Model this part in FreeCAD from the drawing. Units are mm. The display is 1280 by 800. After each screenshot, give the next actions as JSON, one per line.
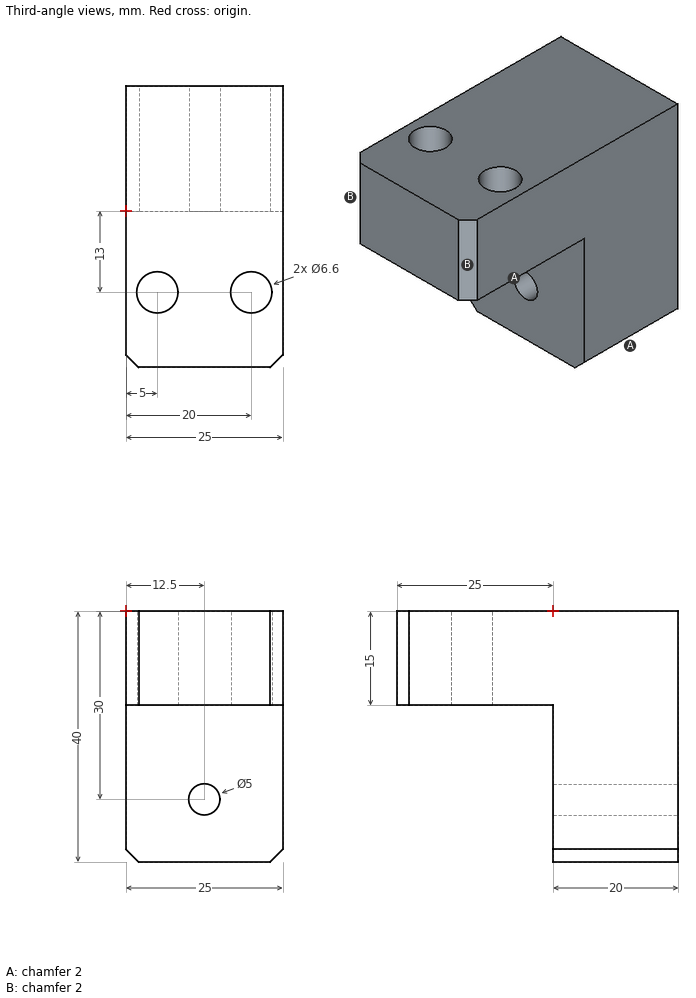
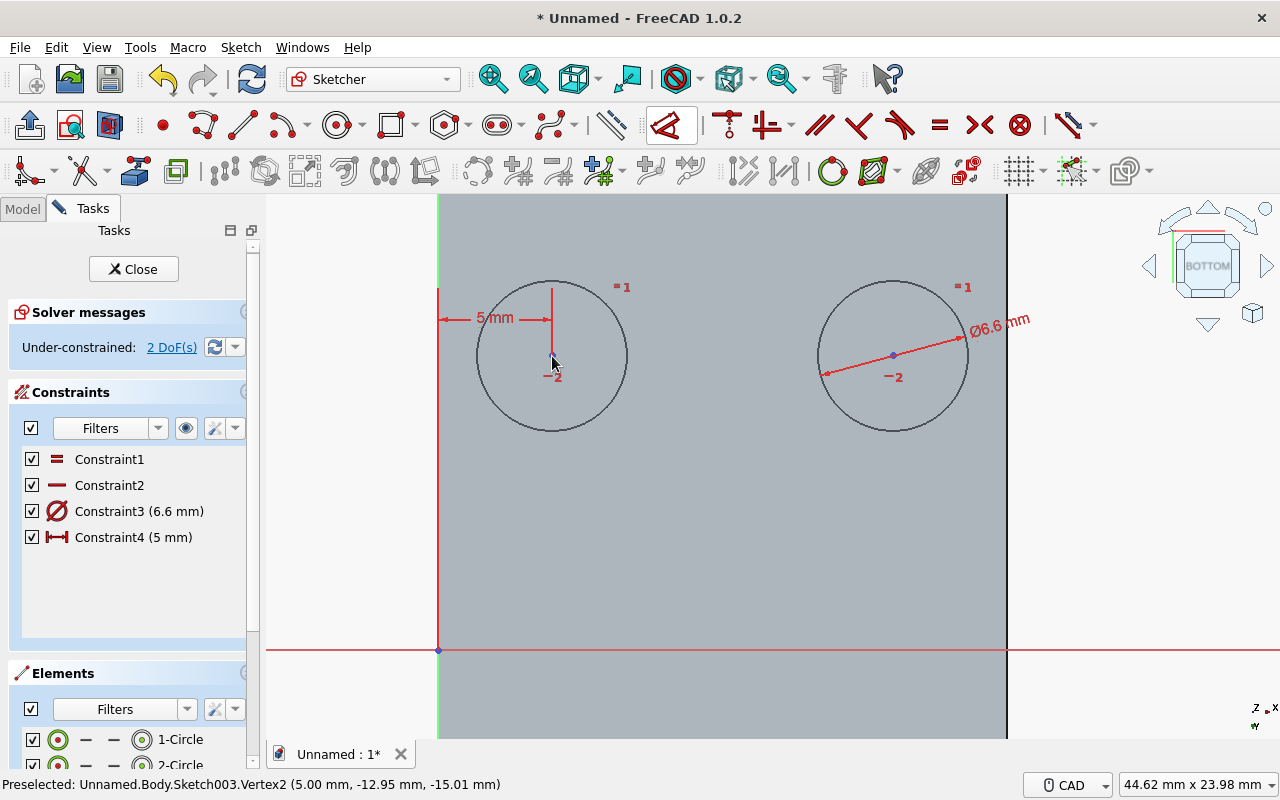
{"action": "left_click", "coordinate": [893, 356]}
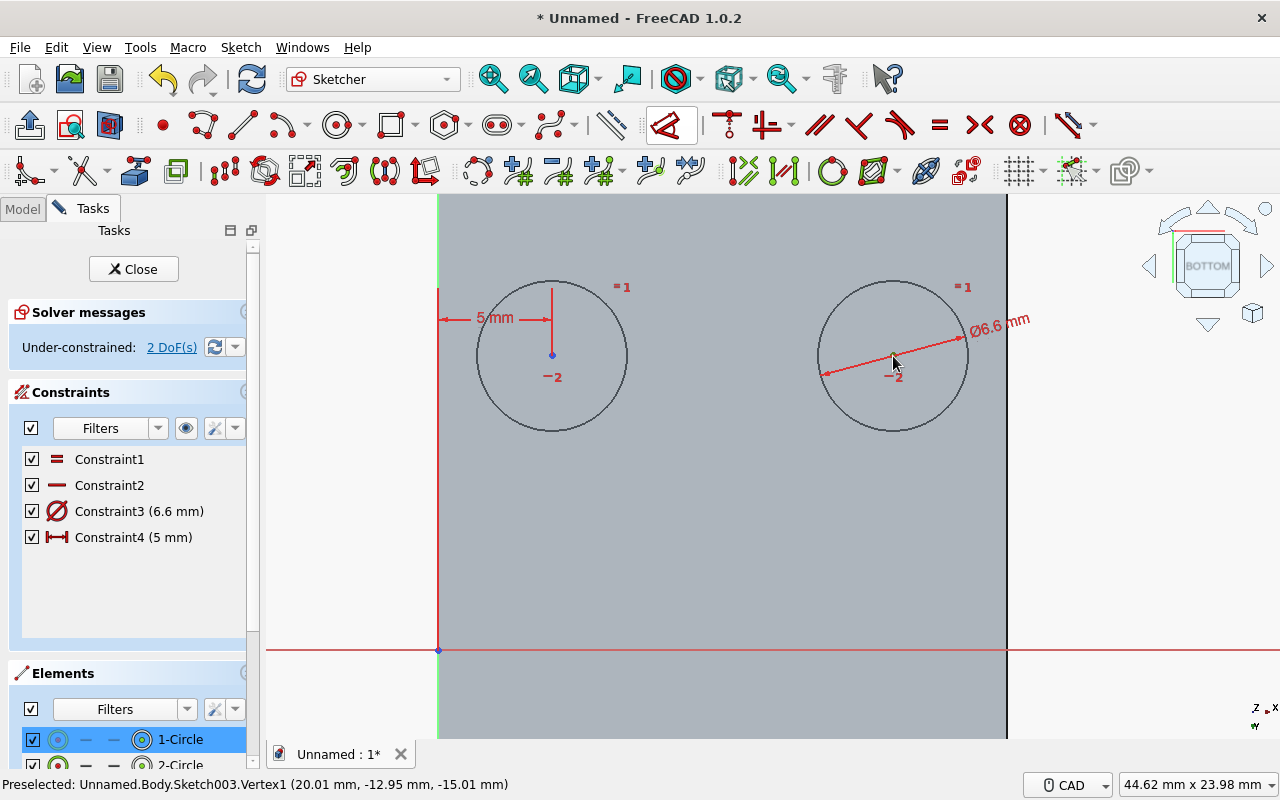
{"action": "key", "text": "l"}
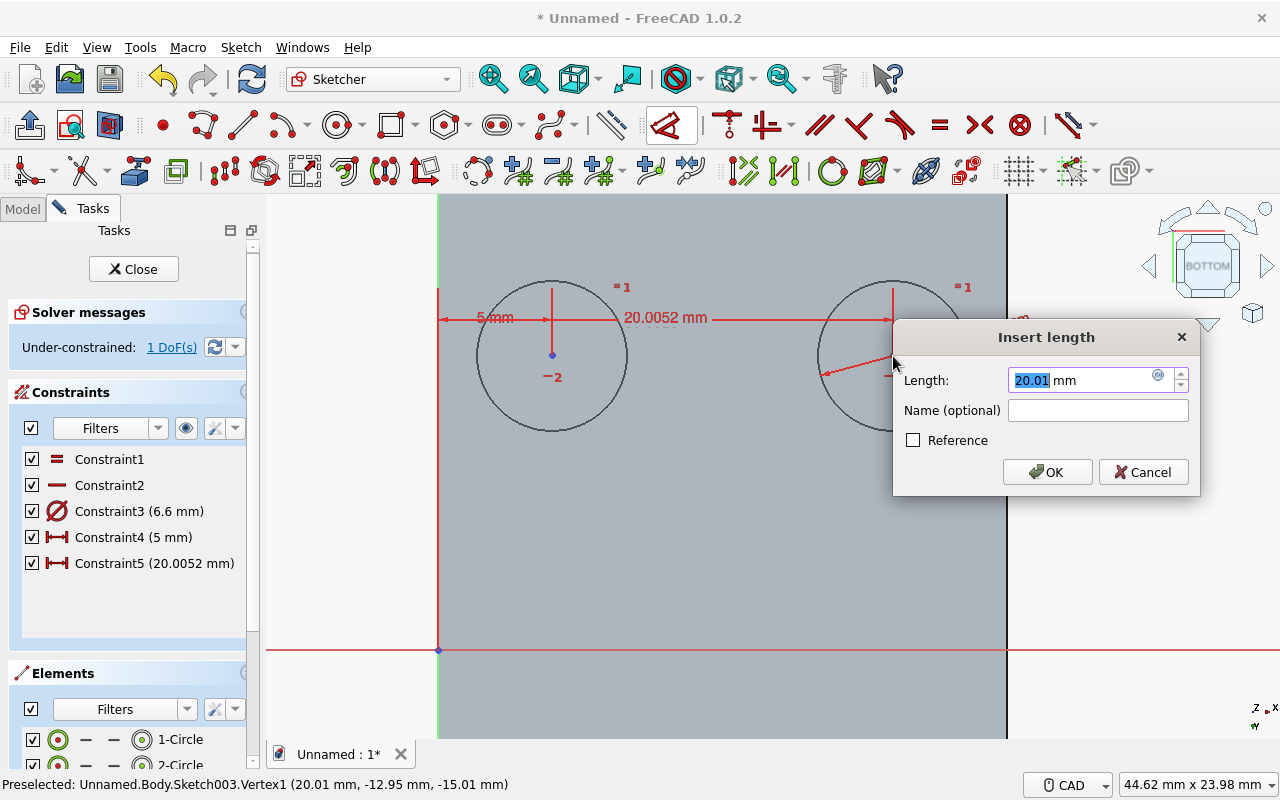
{"action": "type", "text": "20"}
{"action": "key", "text": "Return"}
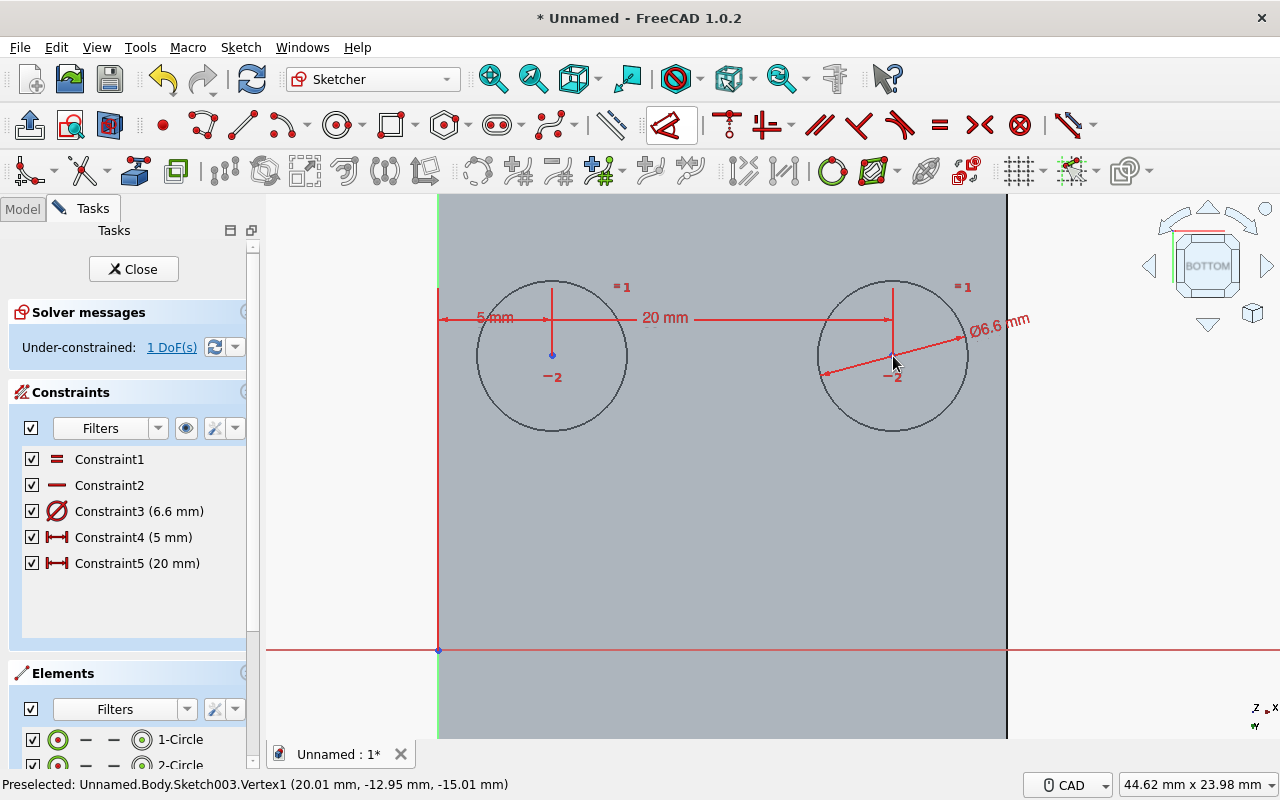
{"action": "left_click", "coordinate": [893, 356]}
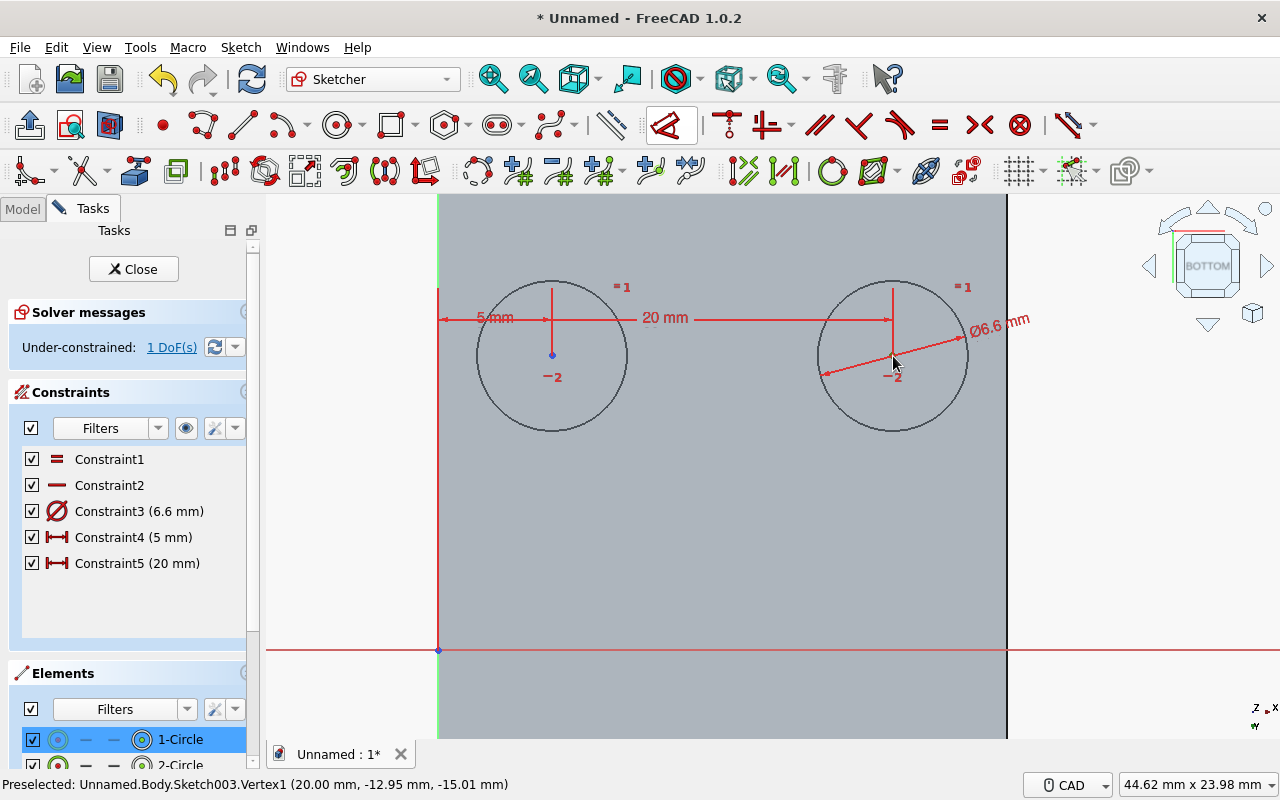
{"action": "key", "text": "i"}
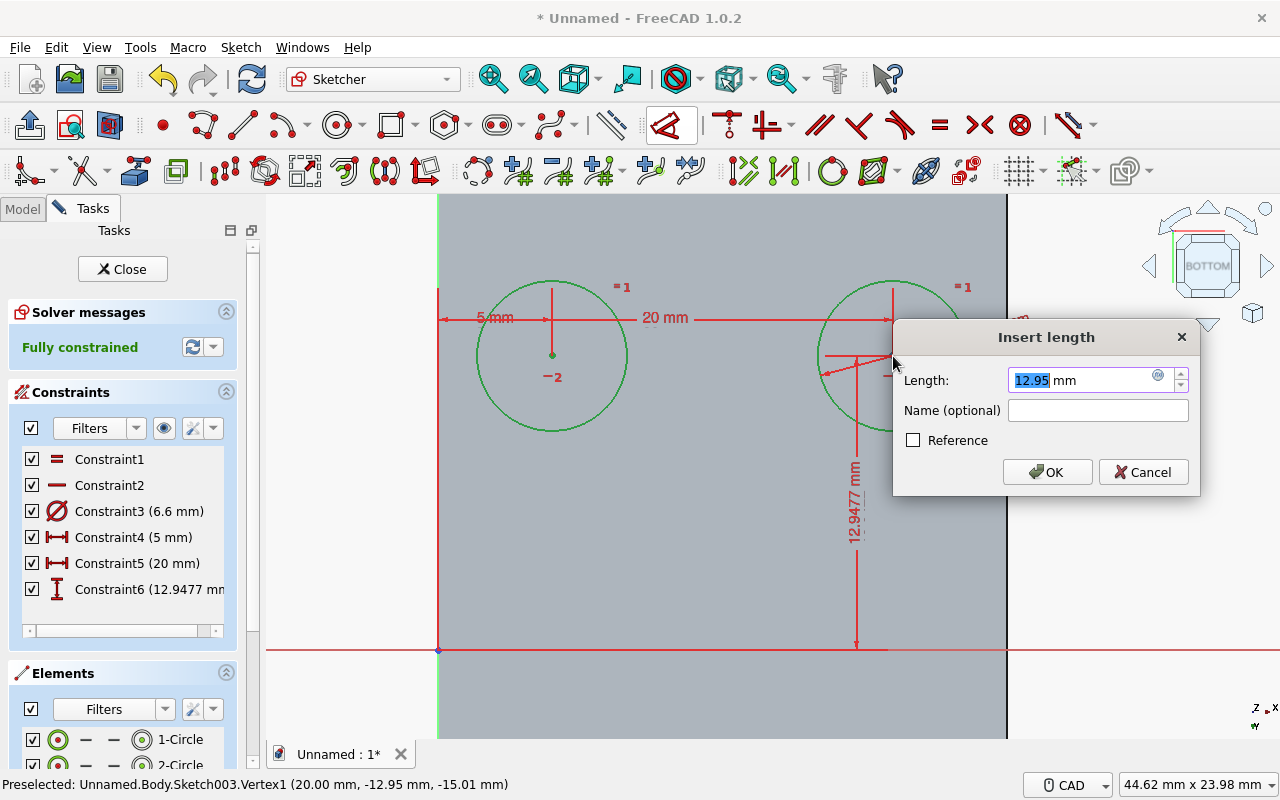
{"action": "type", "text": "13"}
{"action": "key", "text": "Return"}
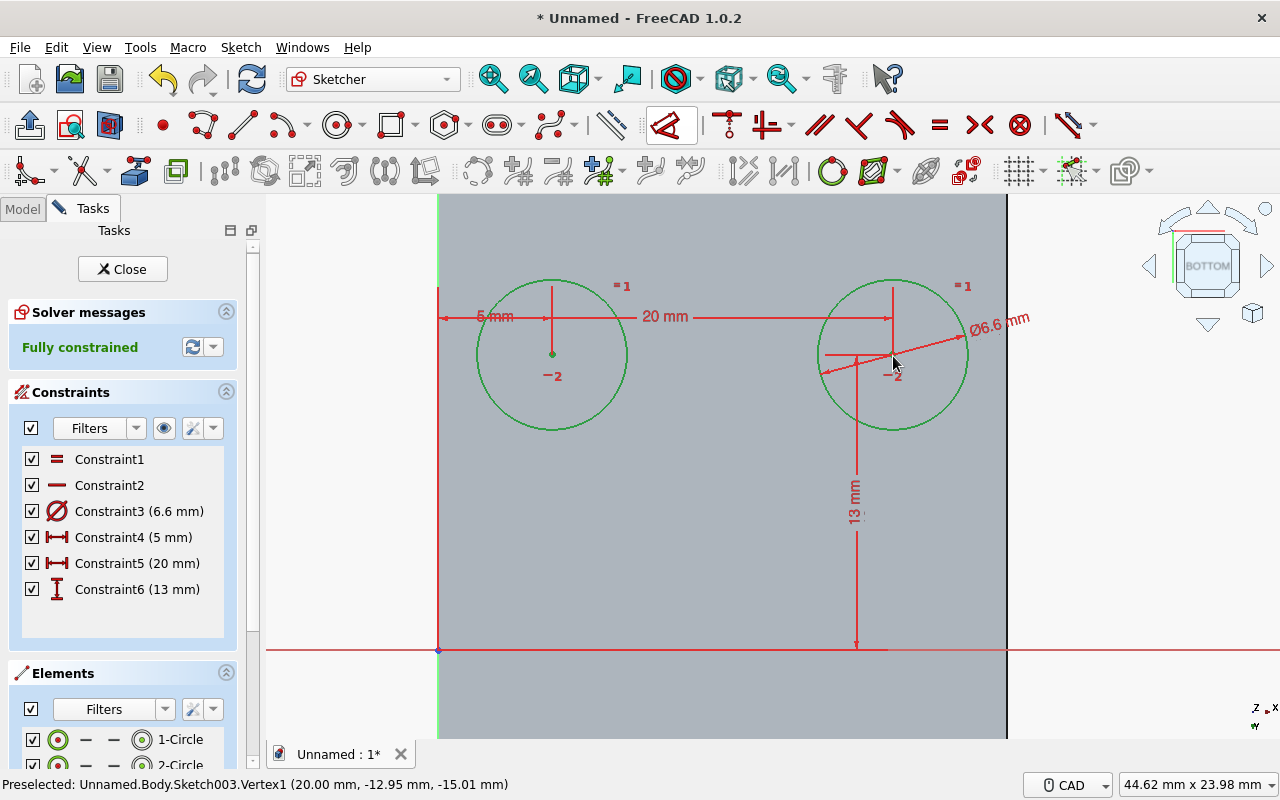
{"action": "left_click", "coordinate": [123, 269]}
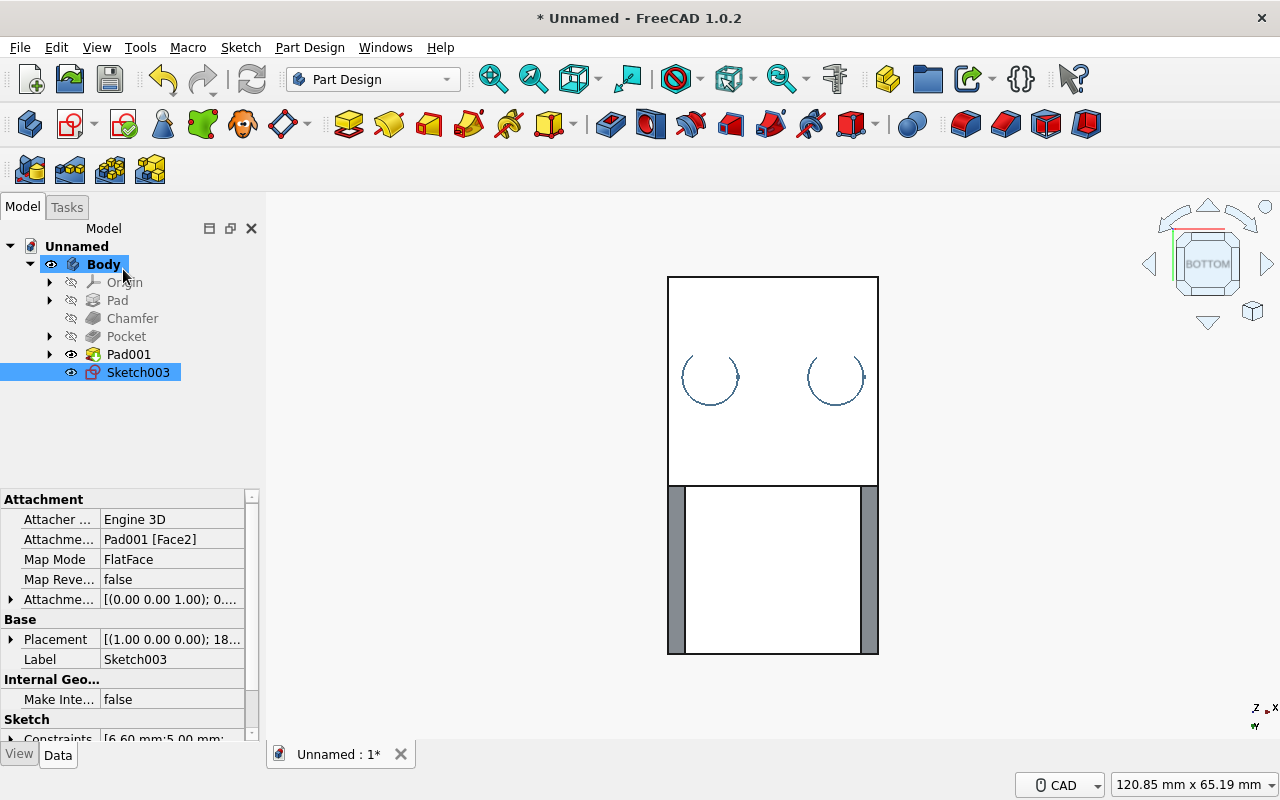
{"action": "left_click", "coordinate": [612, 124]}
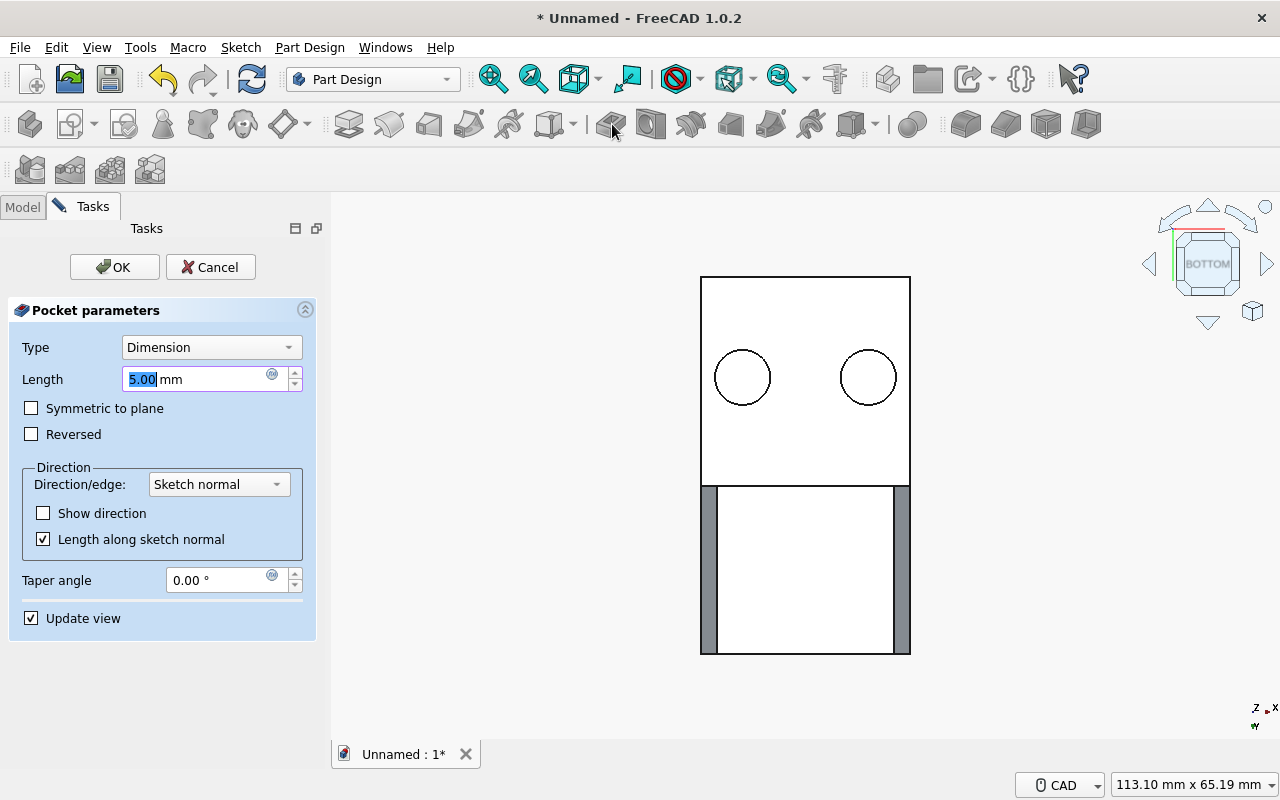
{"action": "left_click", "coordinate": [212, 348]}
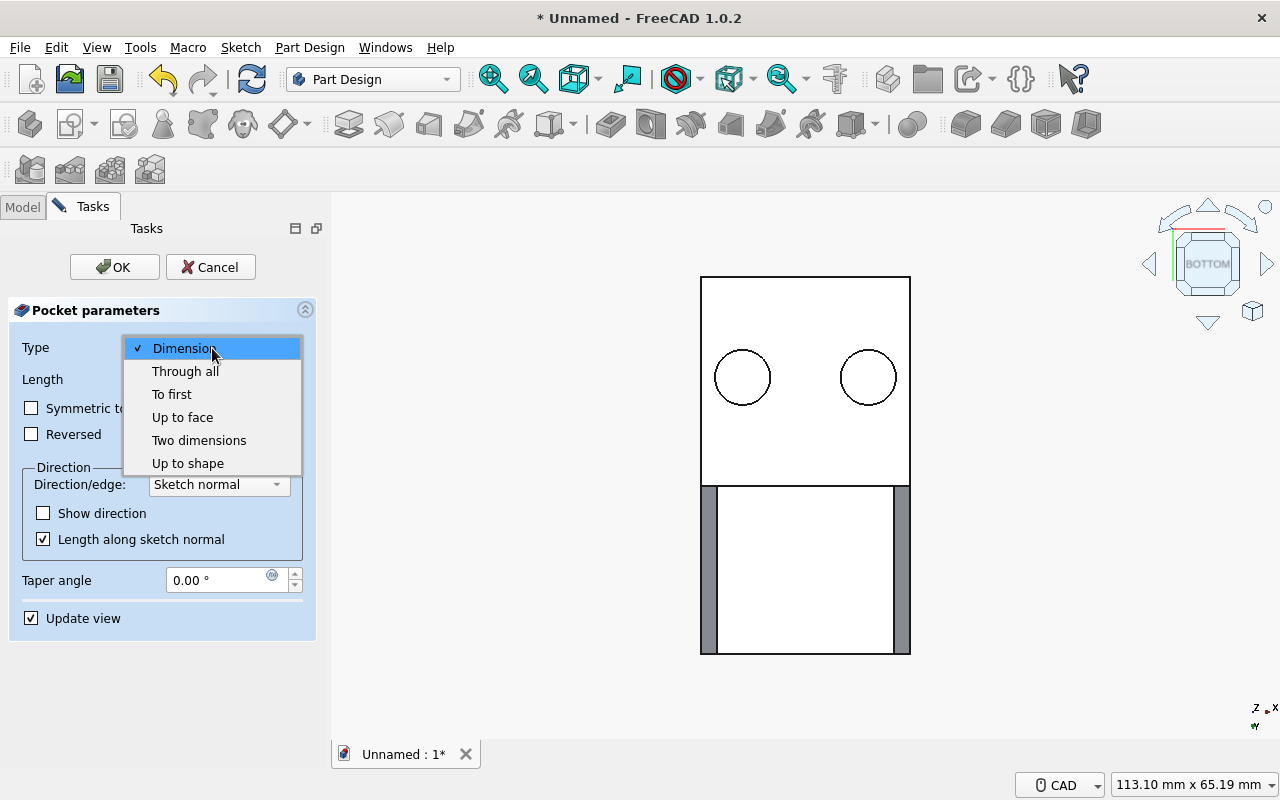
{"action": "left_click", "coordinate": [212, 372]}